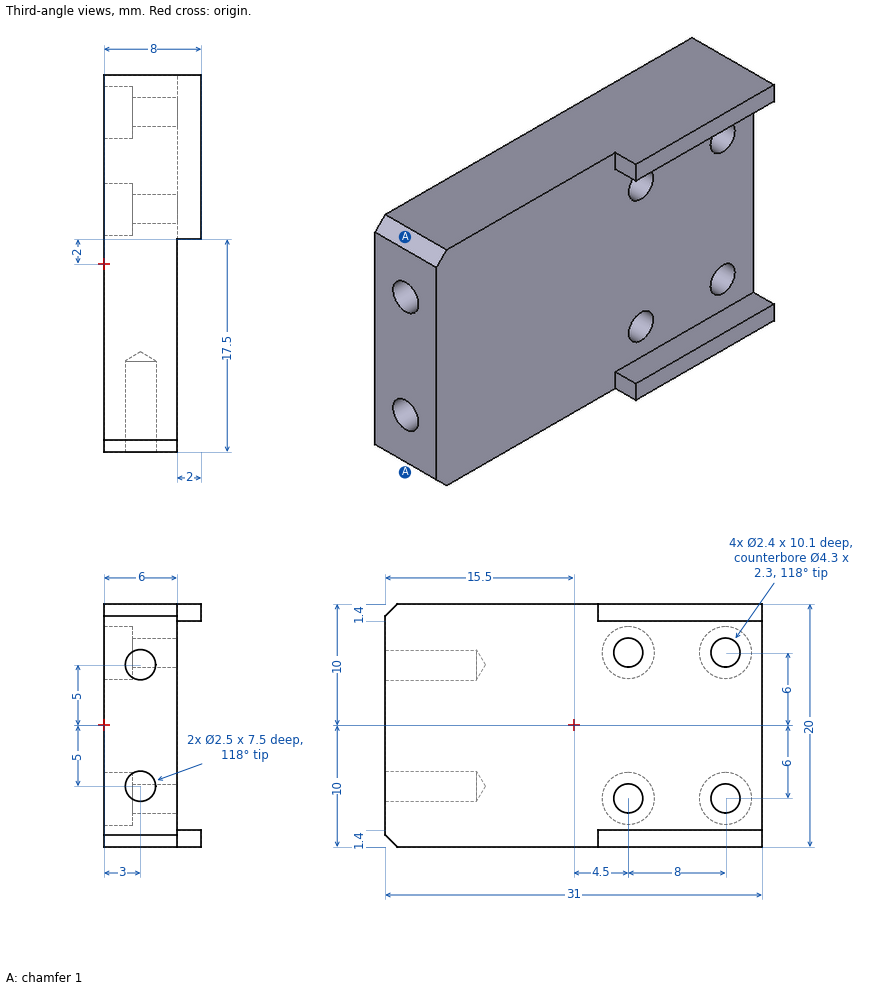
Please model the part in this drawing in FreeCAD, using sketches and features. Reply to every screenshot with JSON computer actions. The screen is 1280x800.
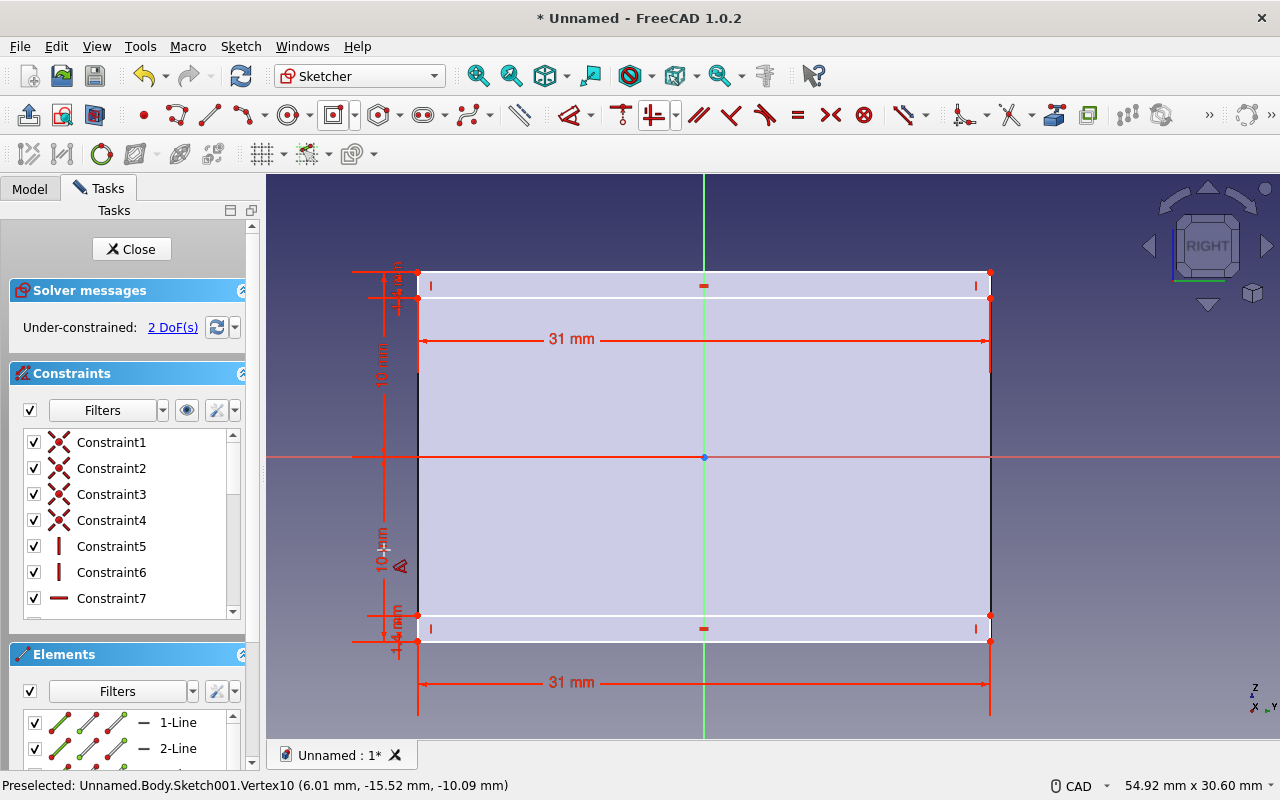
{"action": "left_click", "coordinate": [418, 272]}
{"action": "left_click", "coordinate": [561, 238]}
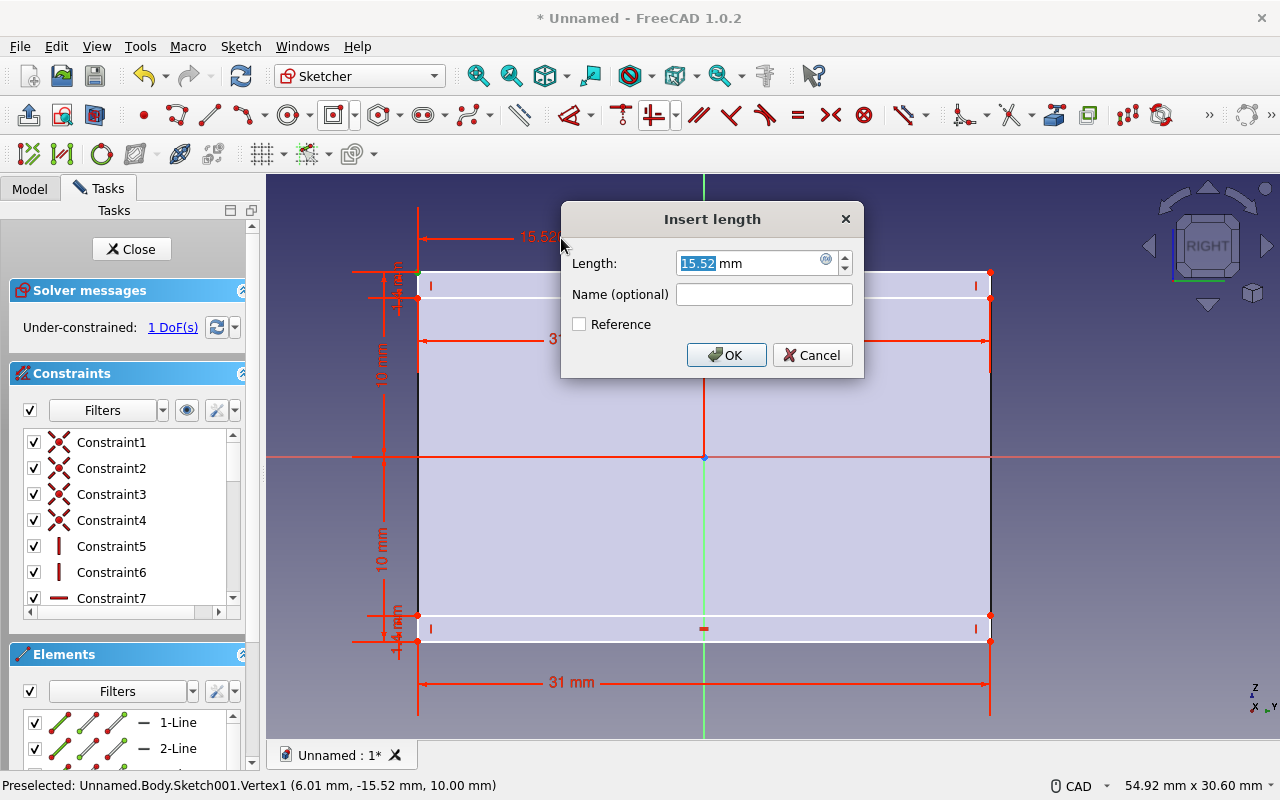
{"action": "type", "text": "15.5"}
{"action": "key", "text": "Return"}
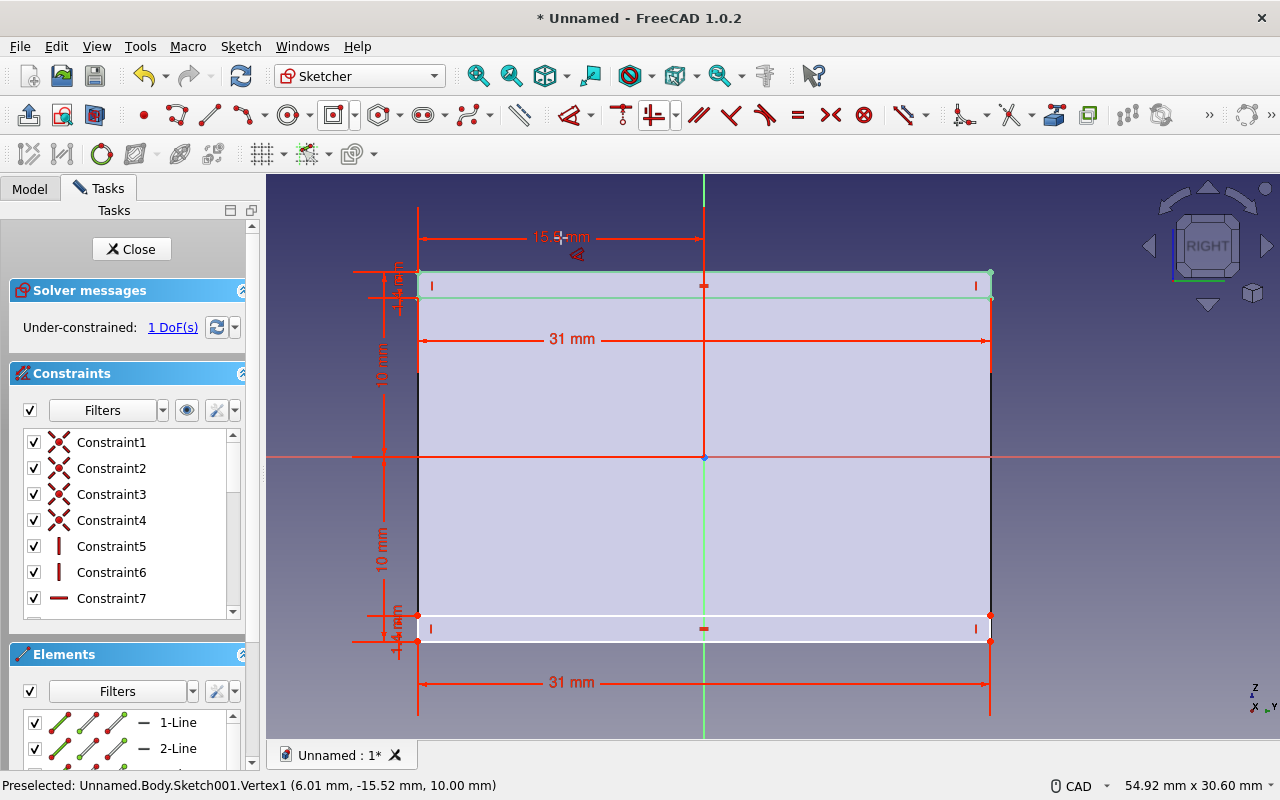
{"action": "left_click", "coordinate": [418, 616]}
{"action": "left_click", "coordinate": [561, 423]}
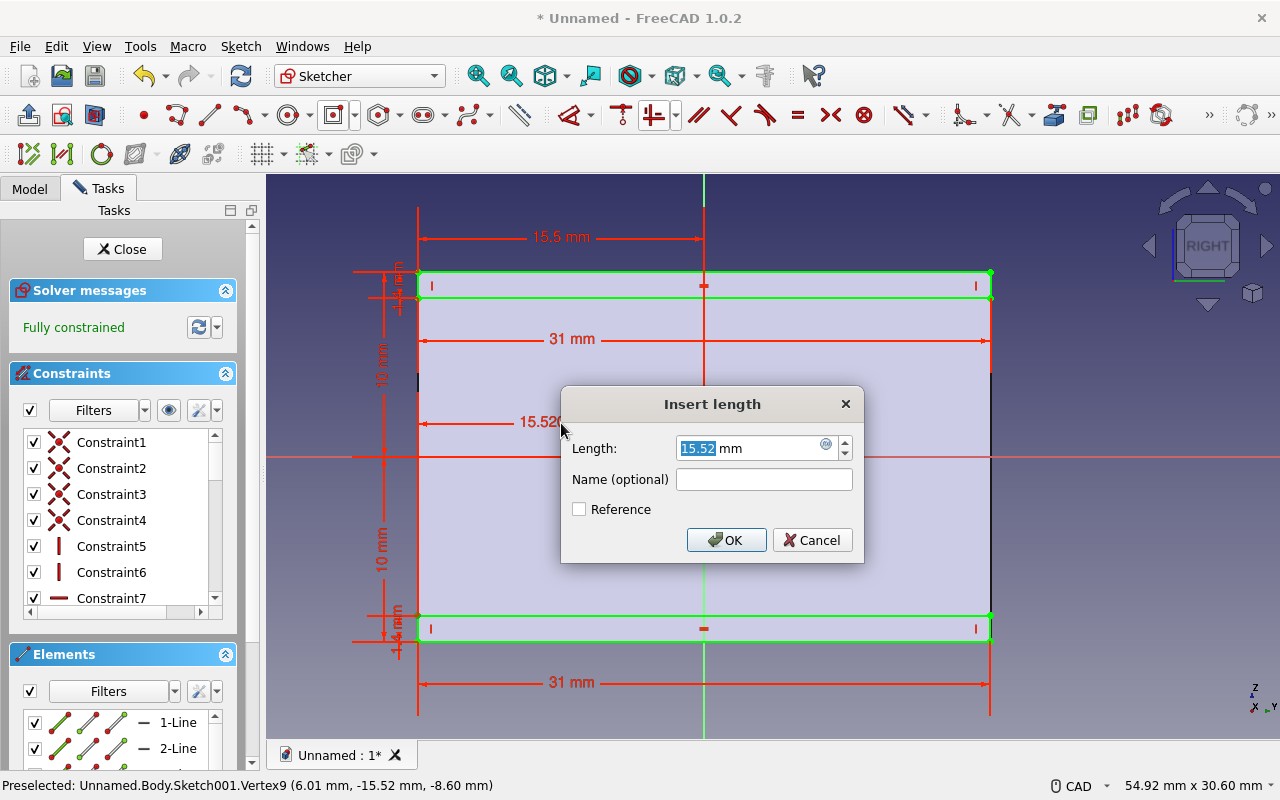
{"action": "type", "text": "15.5"}
{"action": "key", "text": "Return"}
{"action": "key", "text": "Escape"}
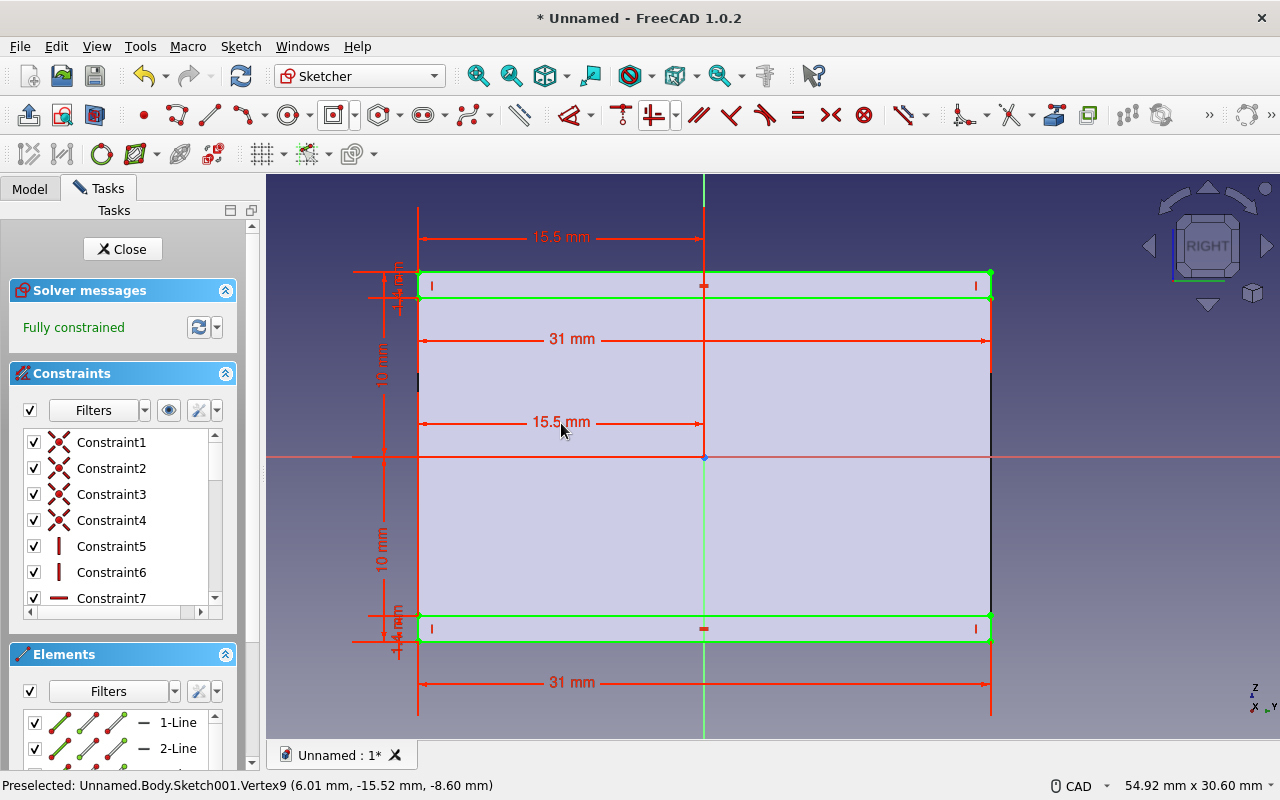
{"action": "left_click", "coordinate": [123, 249]}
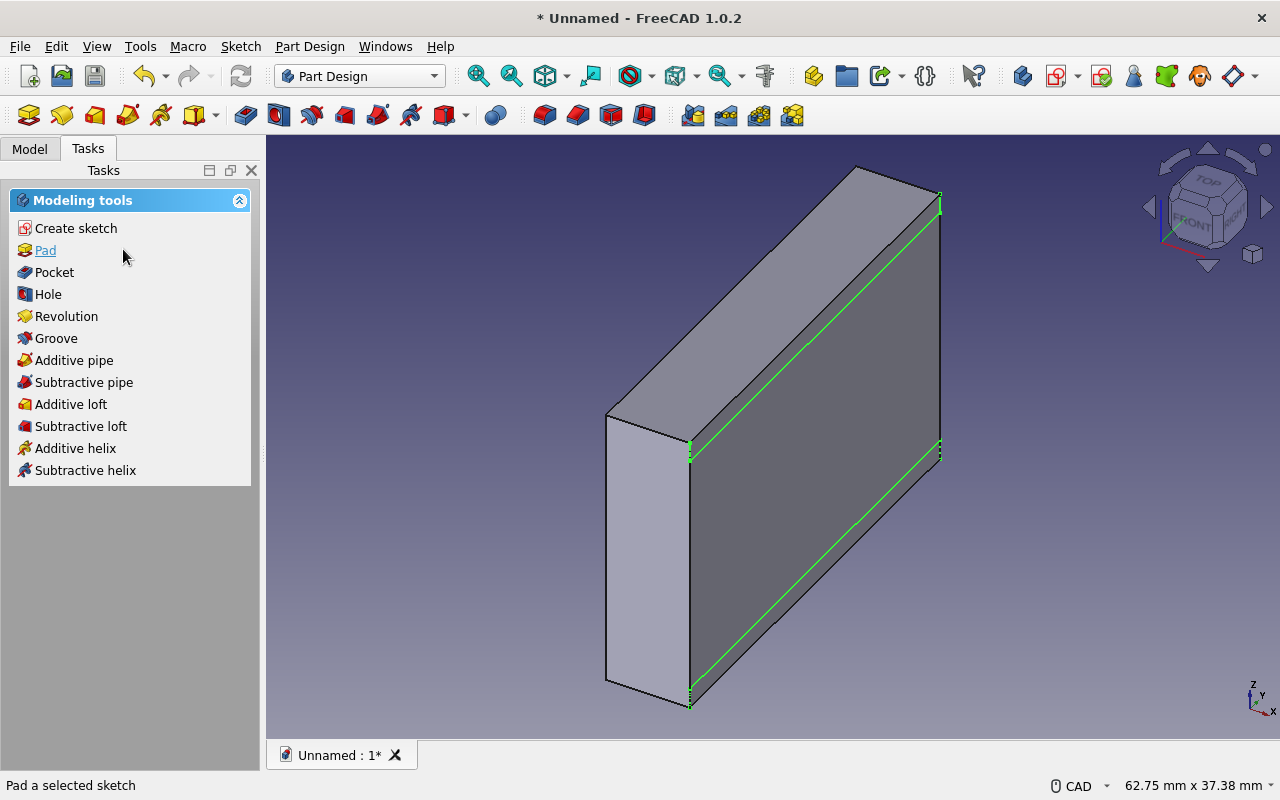
{"action": "left_click", "coordinate": [29, 116]}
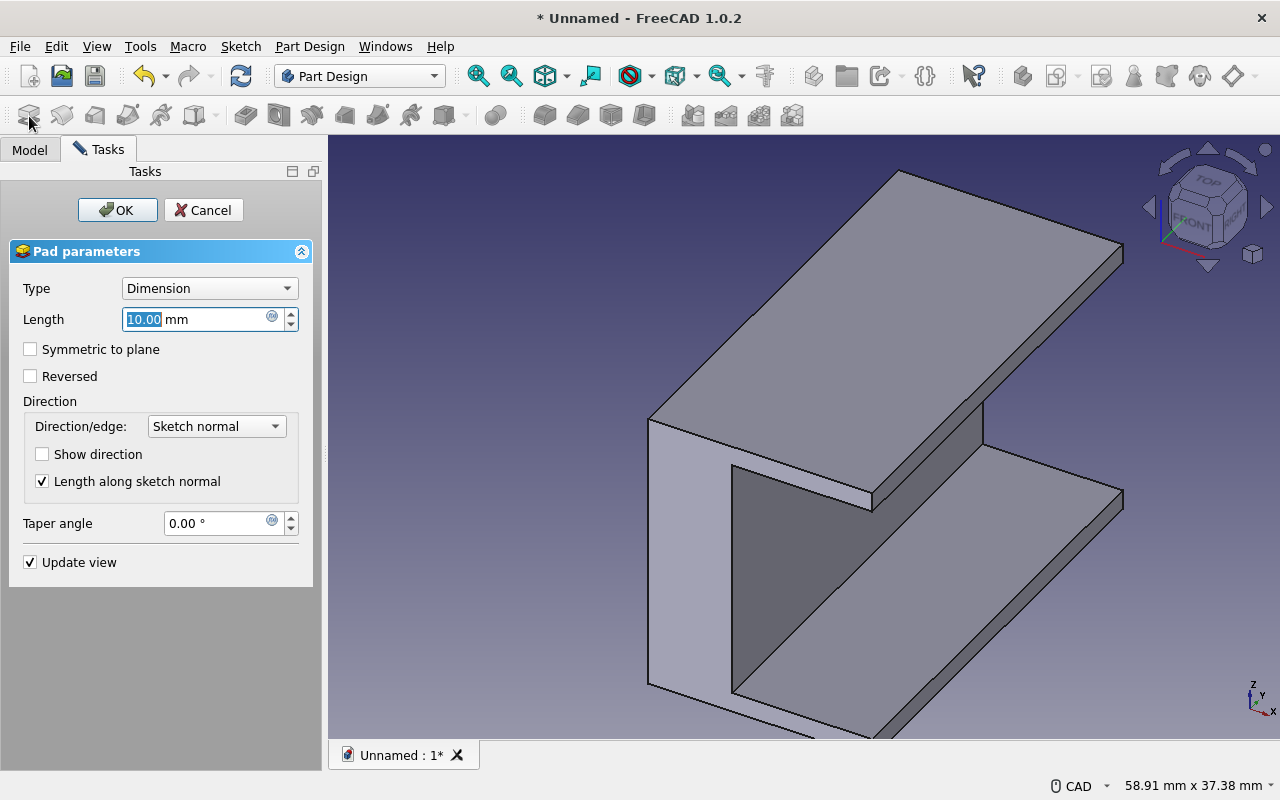
{"action": "type", "text": "2"}
{"action": "key", "text": "Tab"}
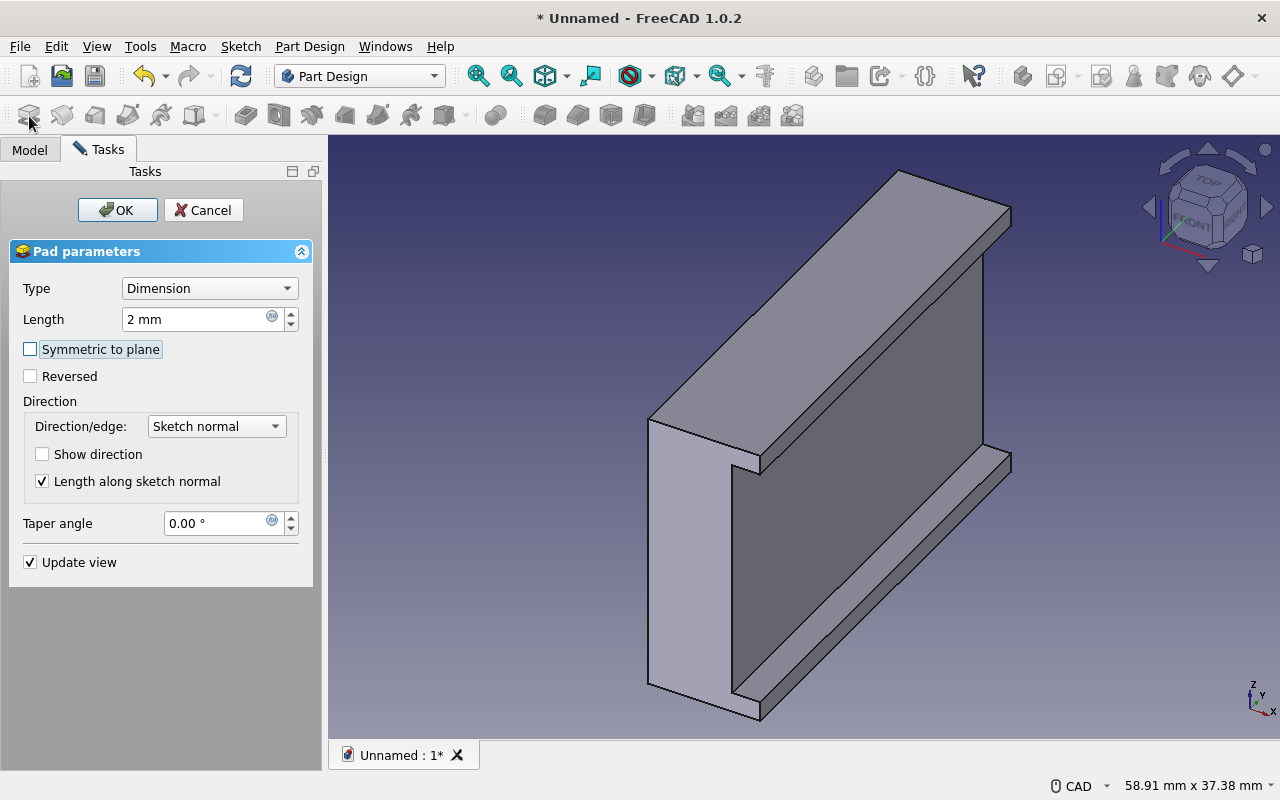
{"action": "left_click", "coordinate": [118, 210]}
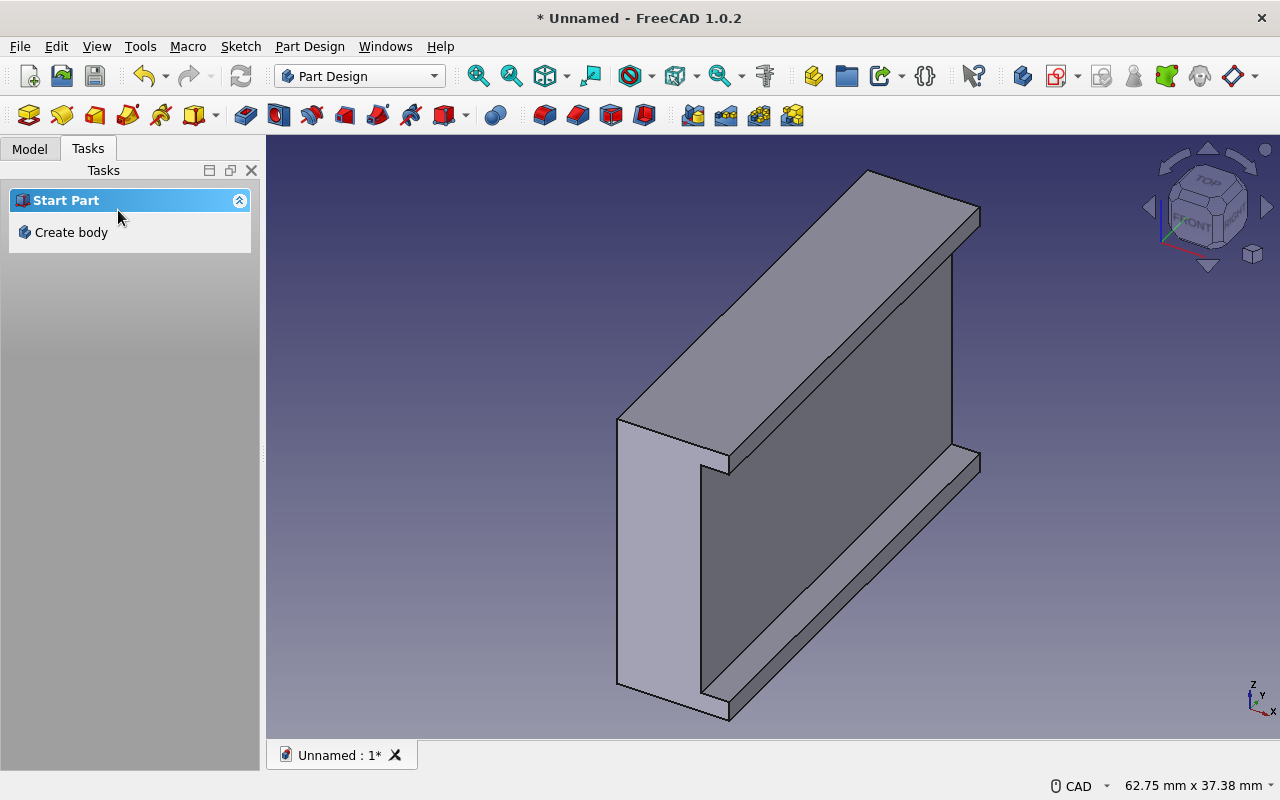
{"action": "left_click", "coordinate": [834, 277]}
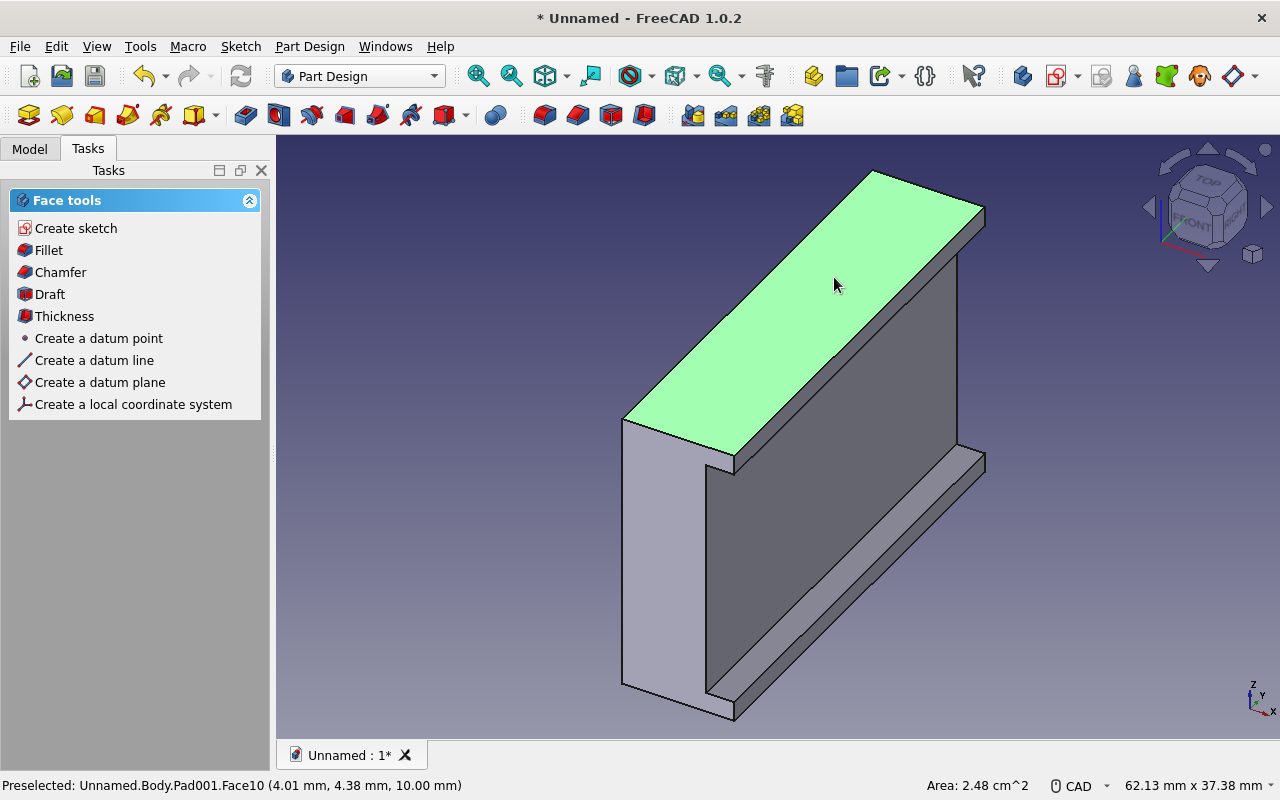
{"action": "left_click", "coordinate": [1056, 76]}